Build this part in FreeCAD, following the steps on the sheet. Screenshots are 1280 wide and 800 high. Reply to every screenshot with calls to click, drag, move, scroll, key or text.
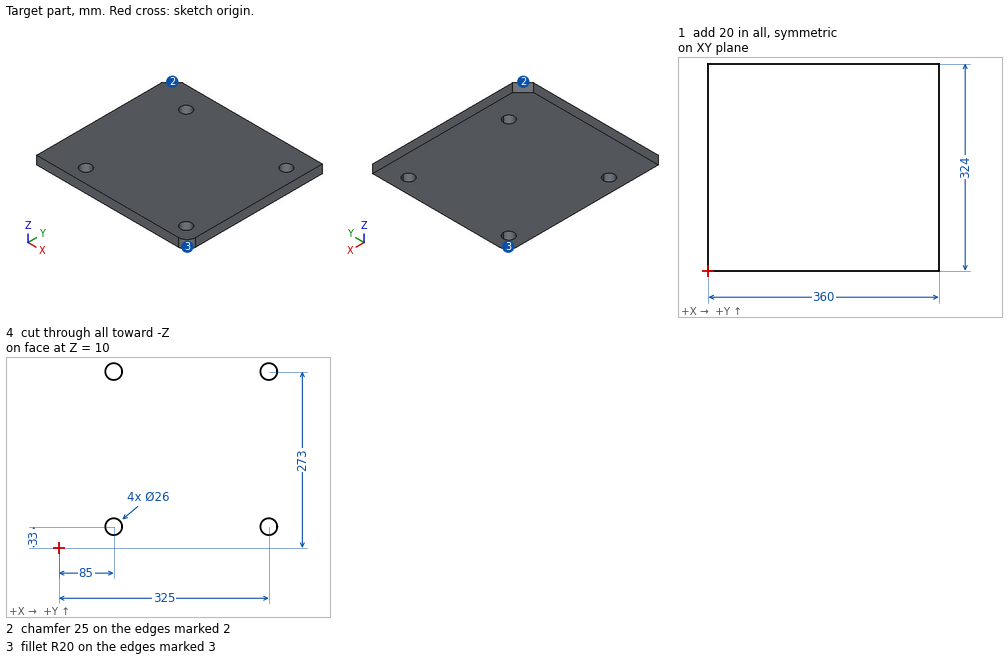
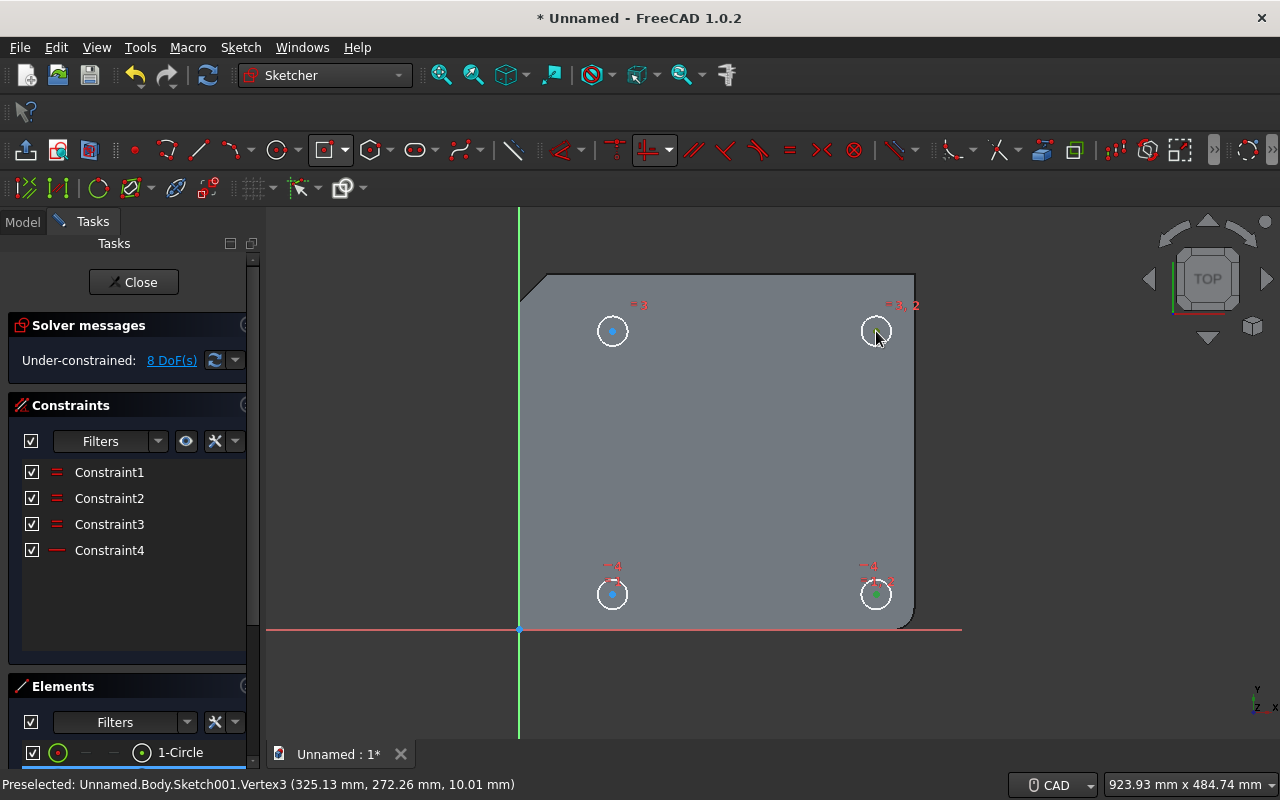
click(672, 150)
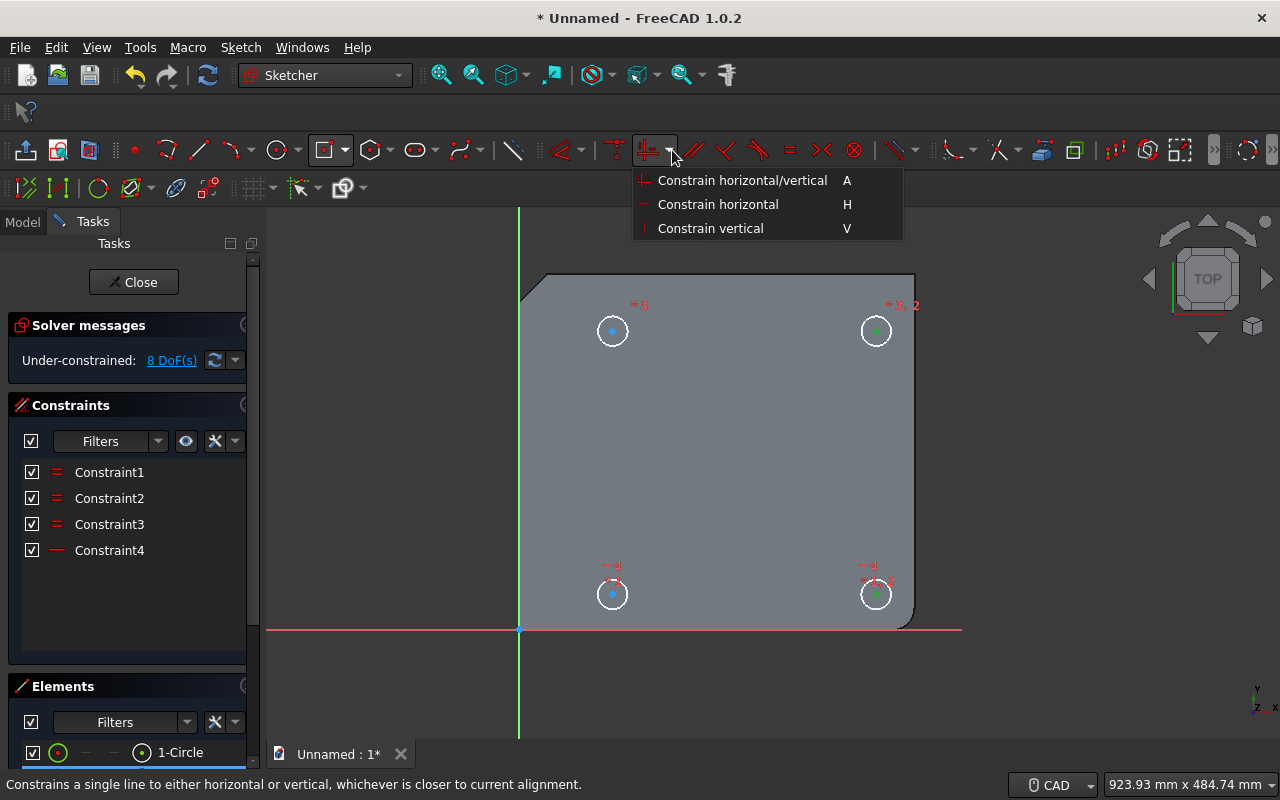
click(768, 228)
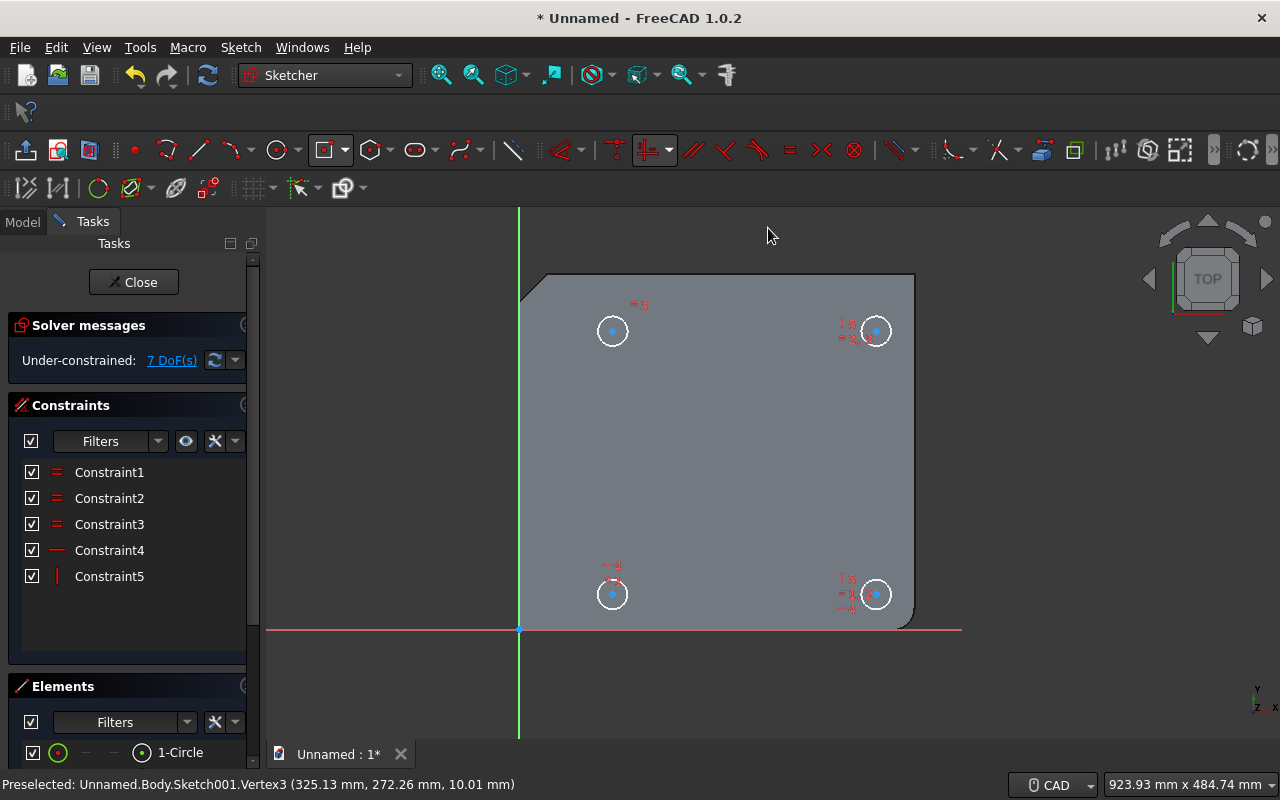
click(613, 595)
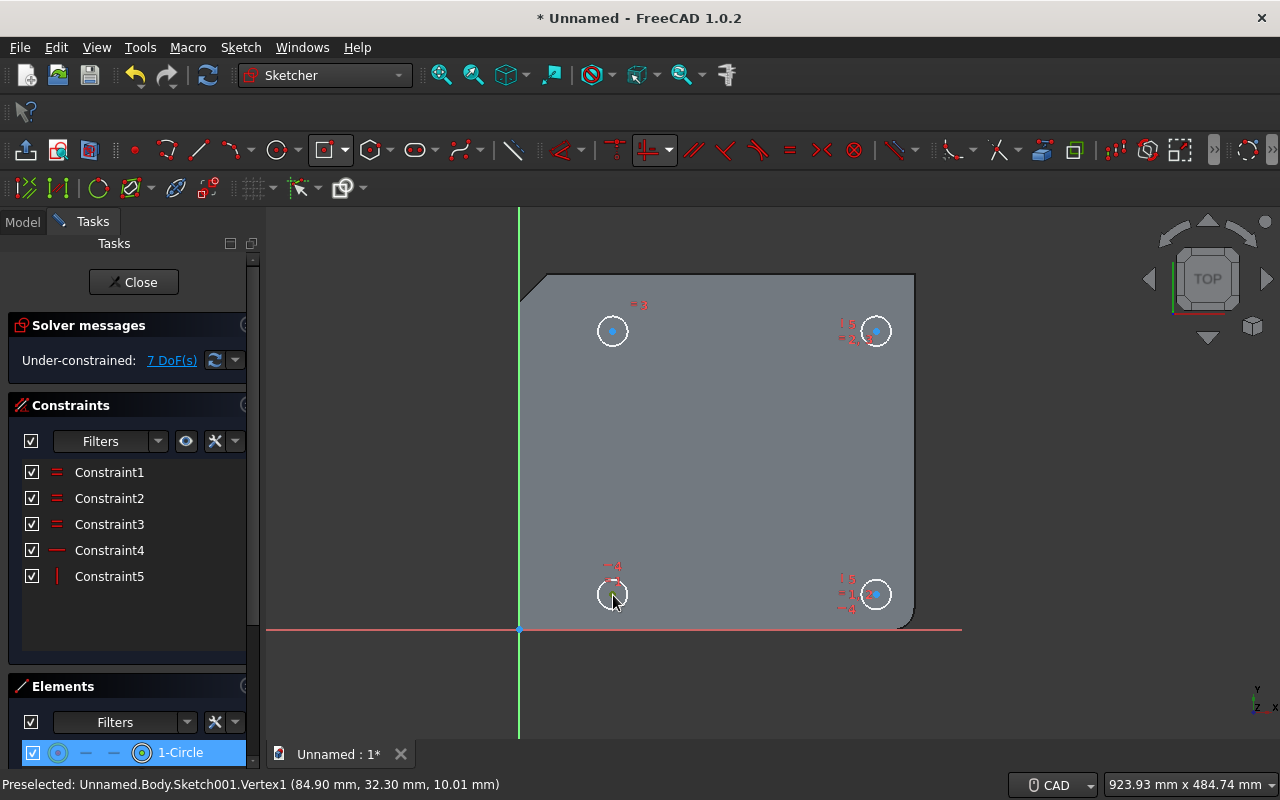
click(613, 331)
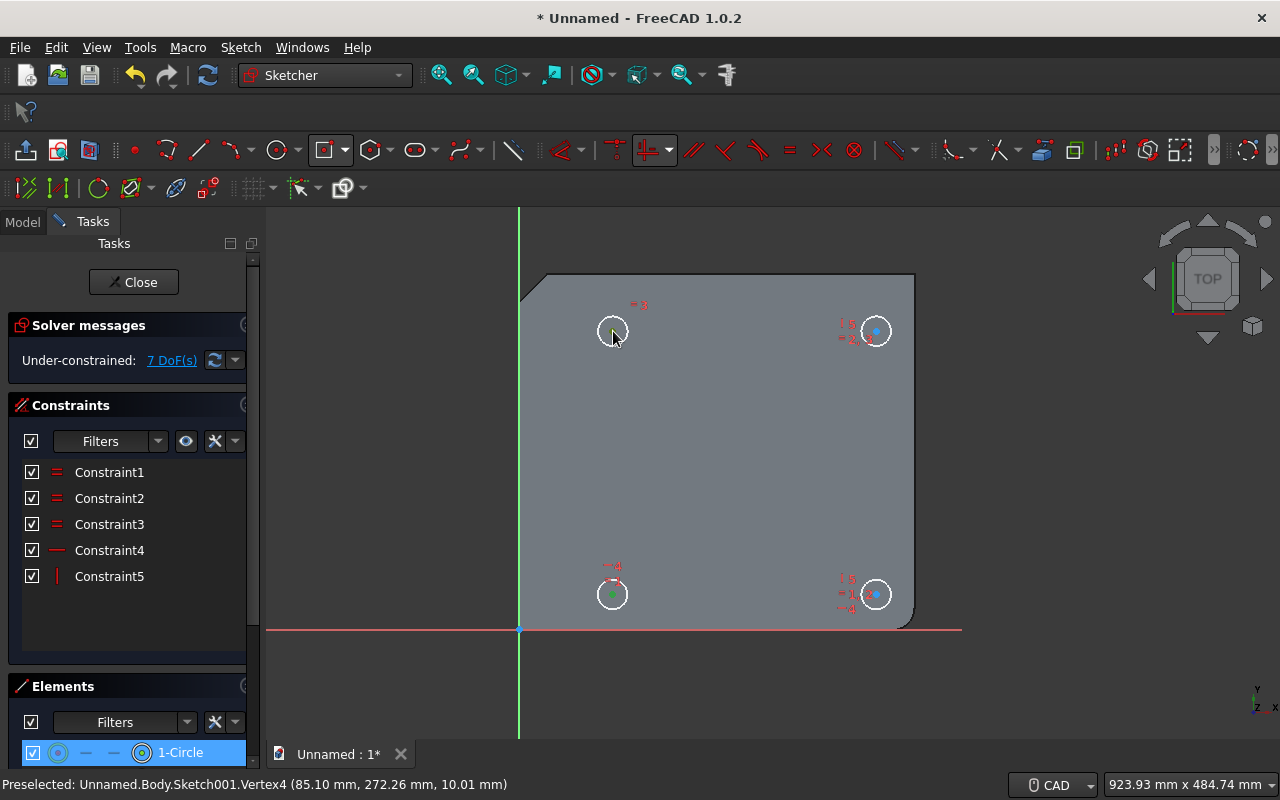
key(v)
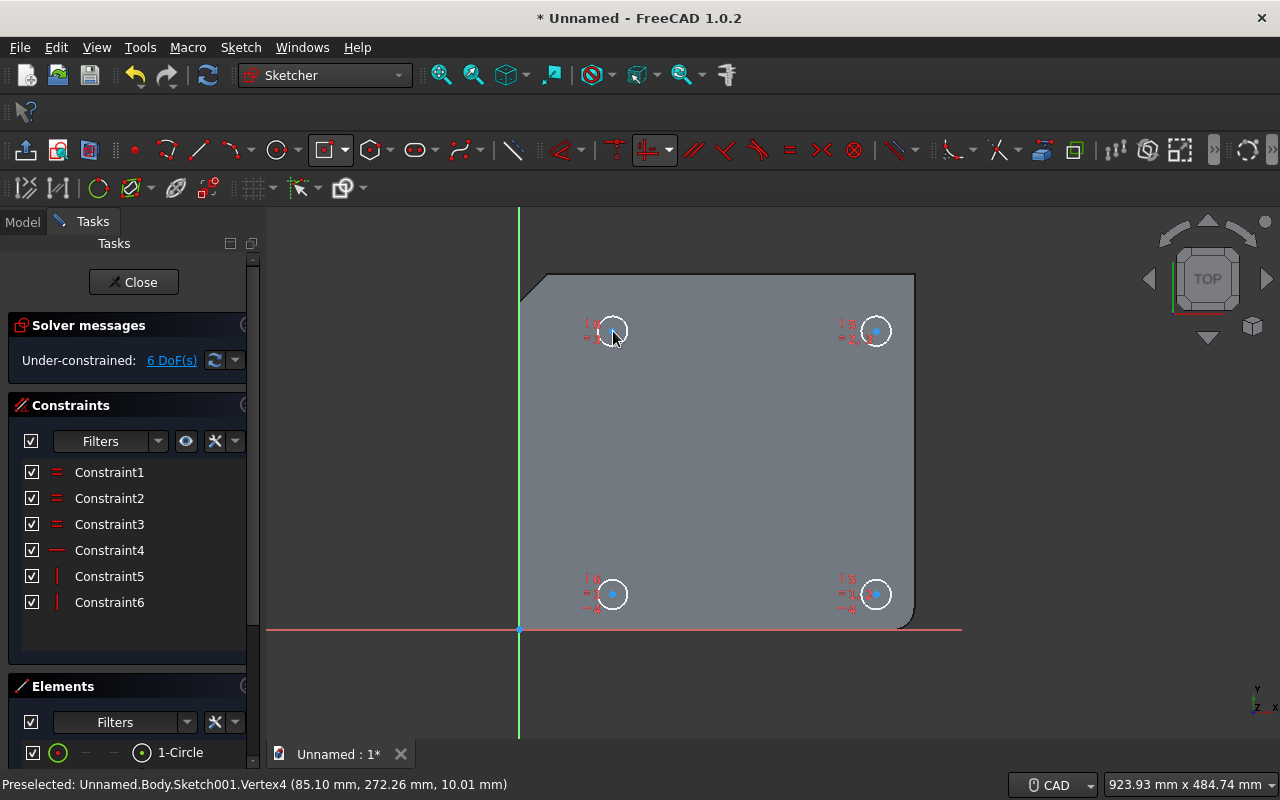
click(876, 331)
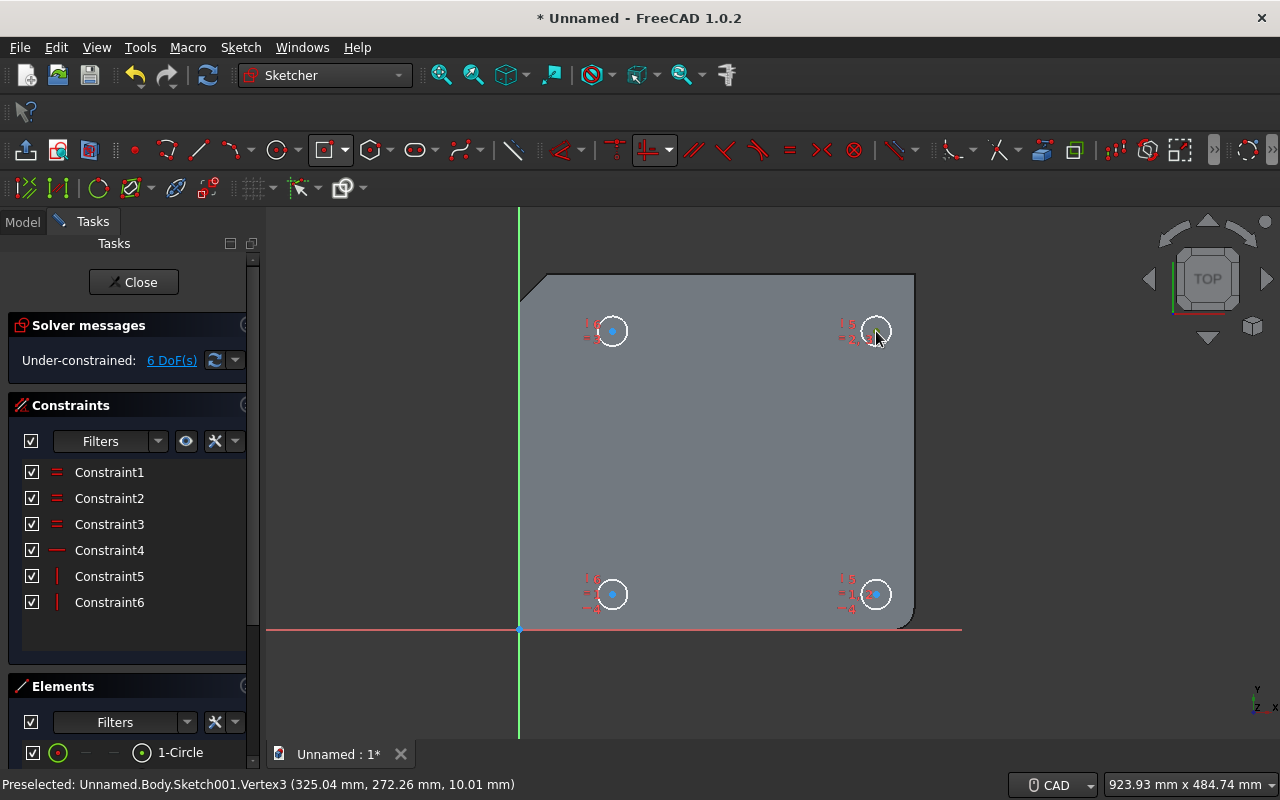
click(613, 331)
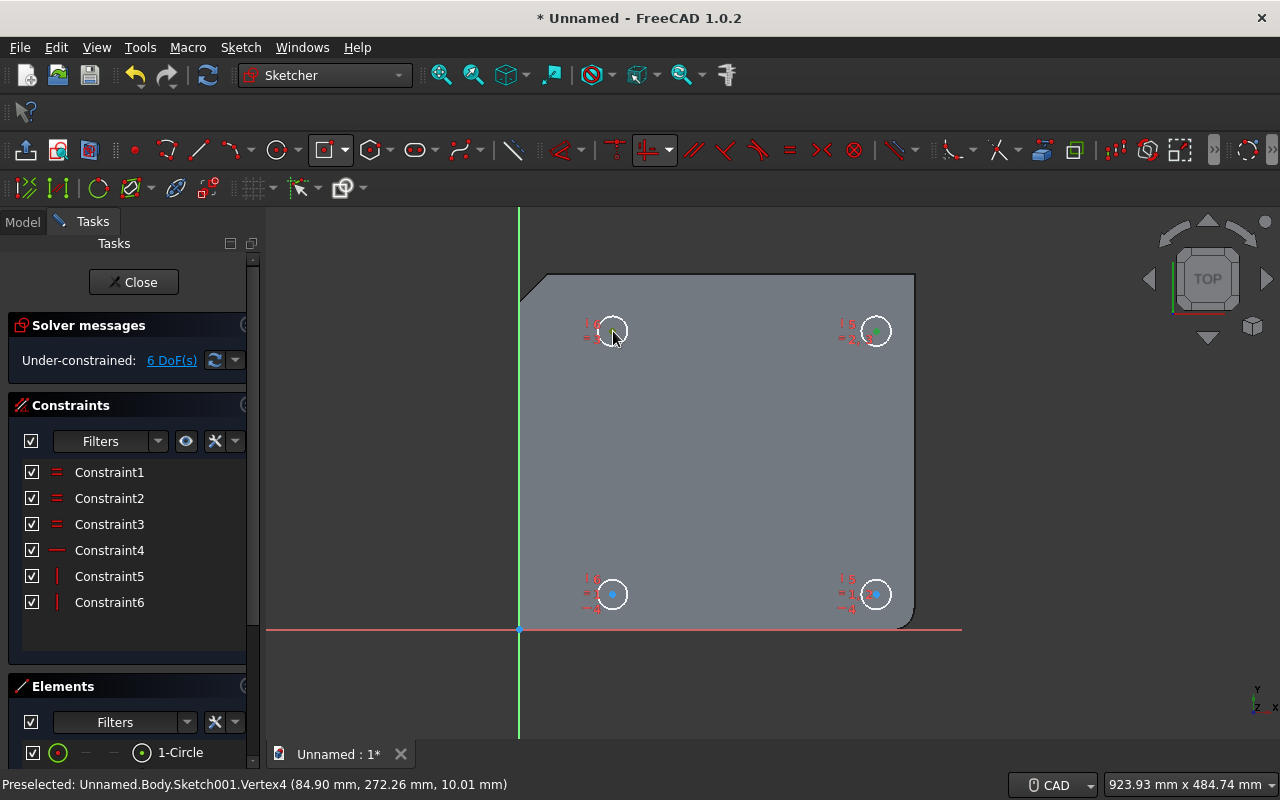
key(h)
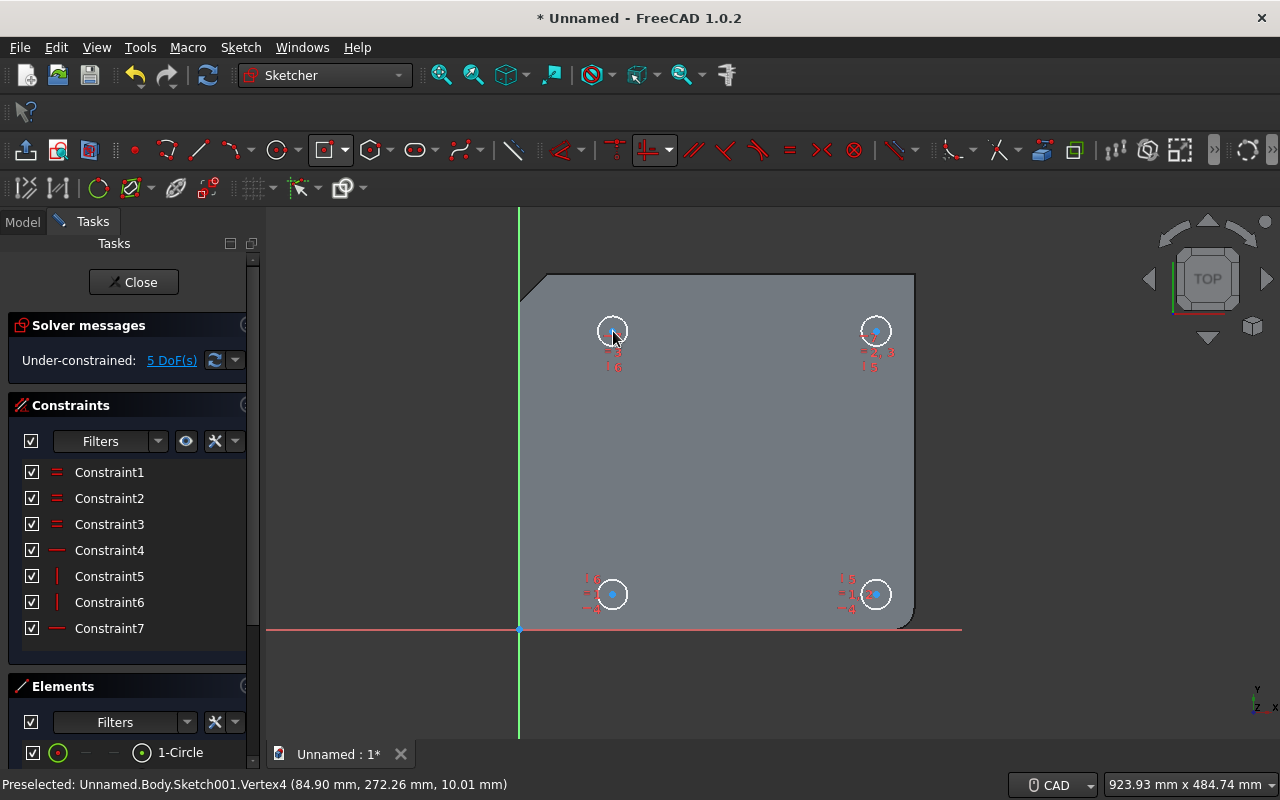
click(560, 150)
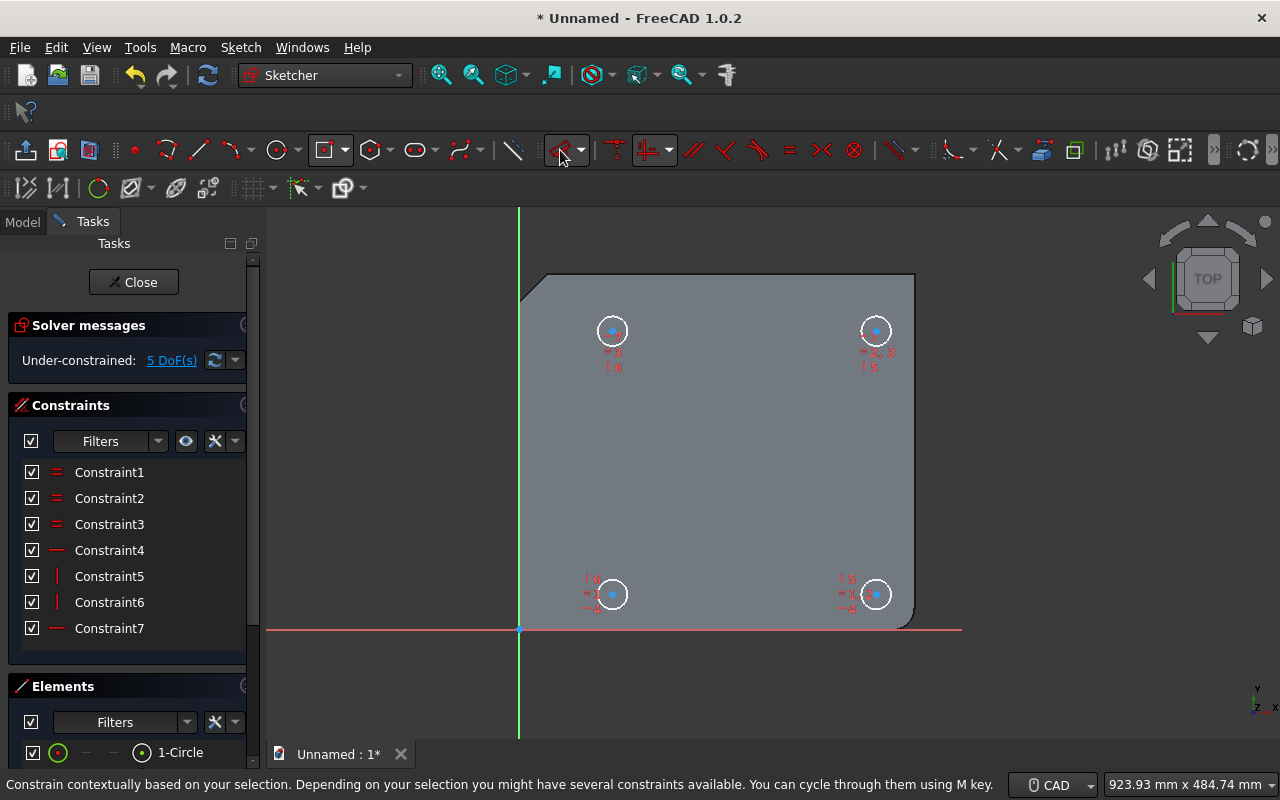
scroll(623, 584, up, 2)